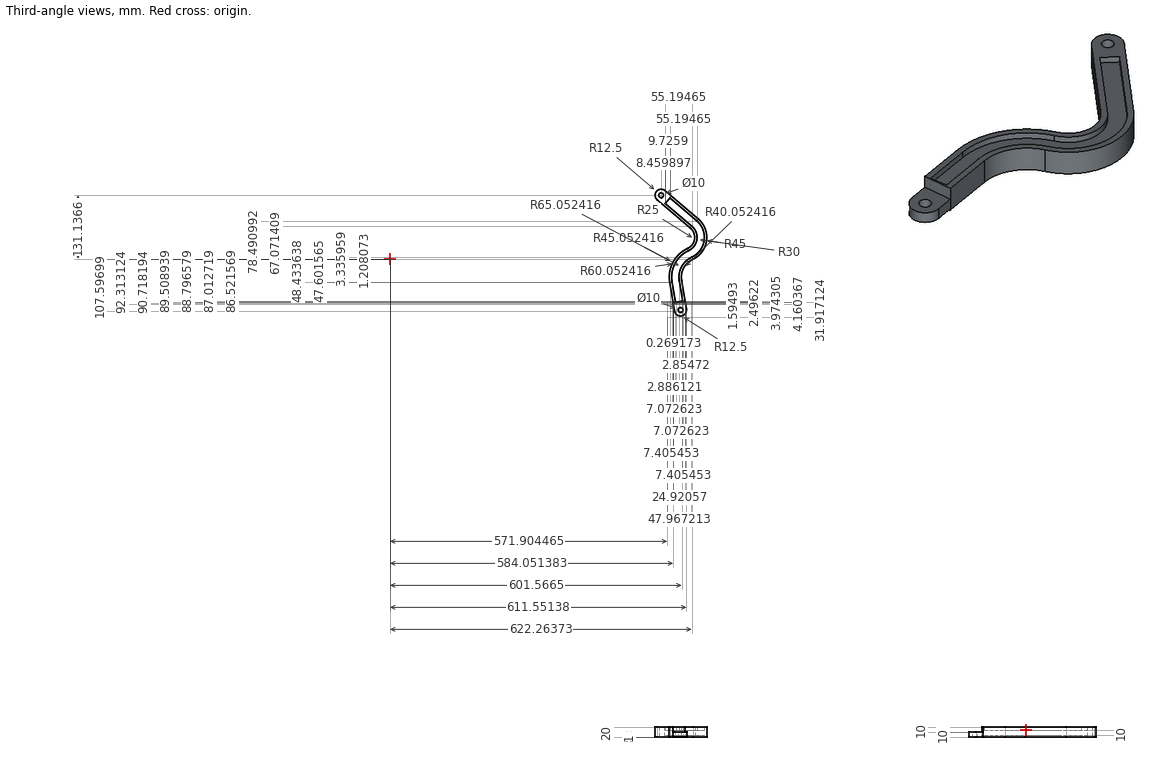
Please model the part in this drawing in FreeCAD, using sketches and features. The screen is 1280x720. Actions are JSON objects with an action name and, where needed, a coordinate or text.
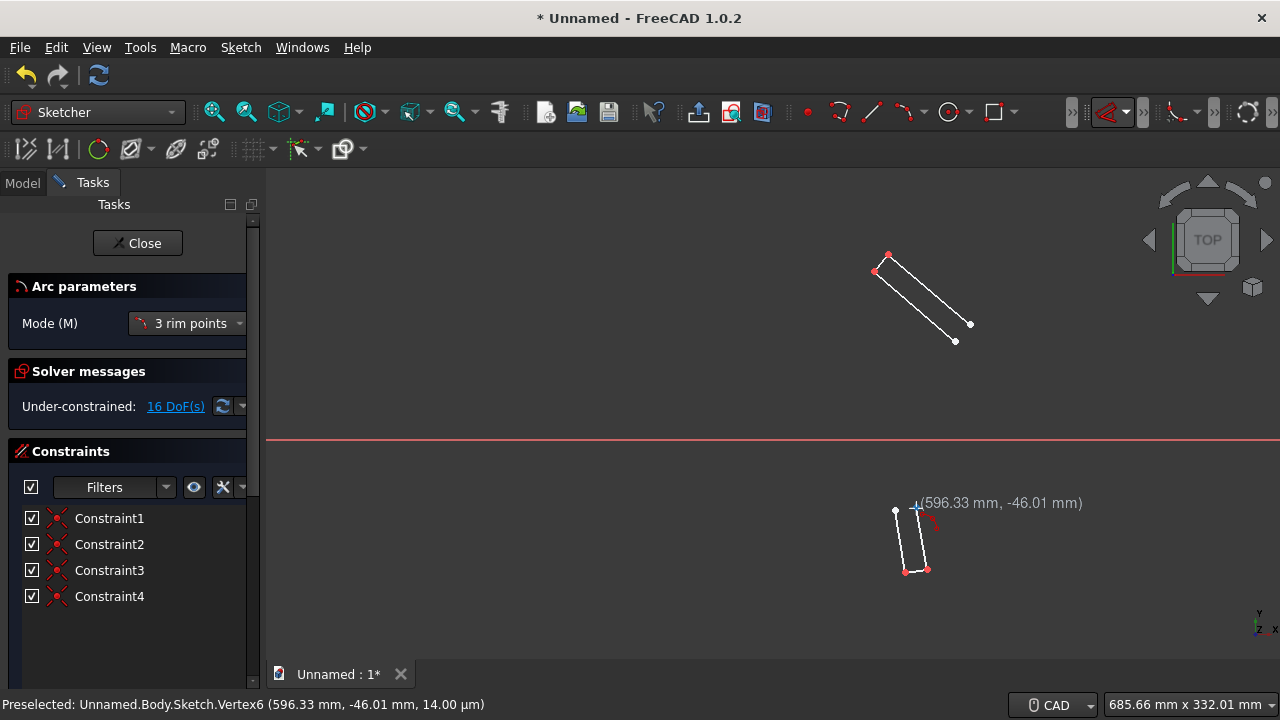
{"action": "scroll", "coordinate": [954, 435], "scroll_direction": "up", "scroll_amount": 6}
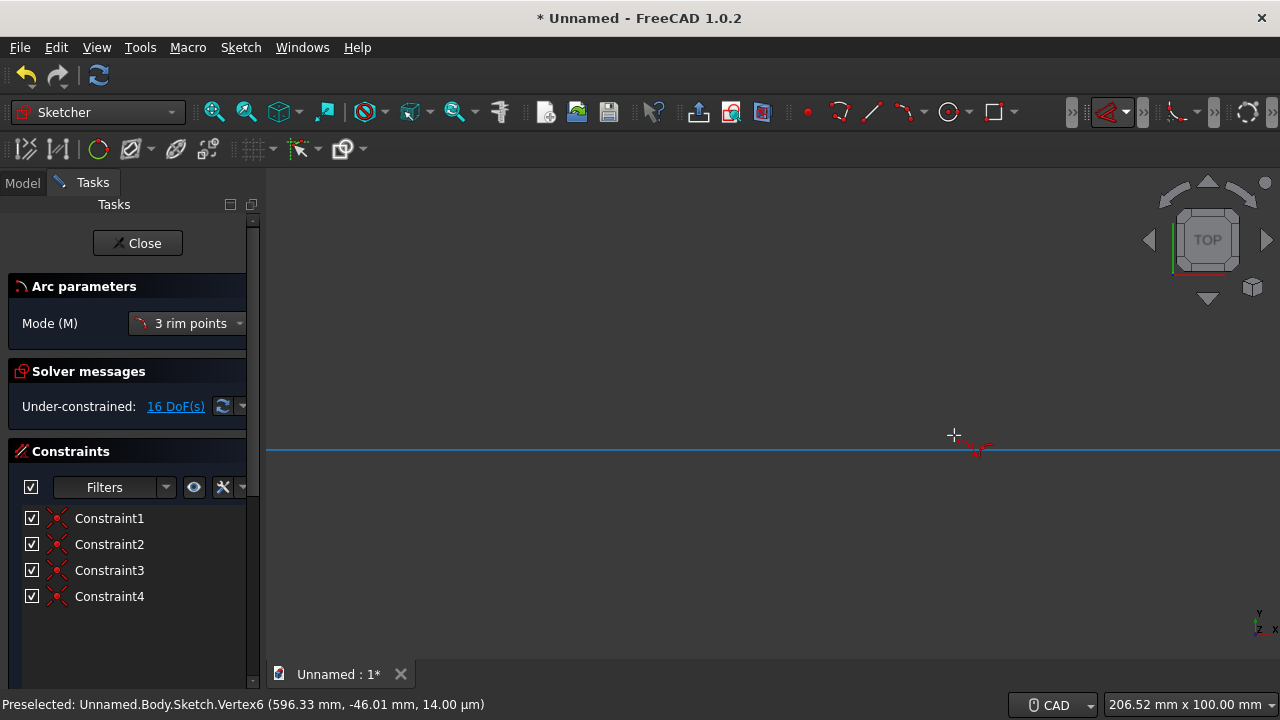
{"action": "left_click", "coordinate": [954, 434]}
{"action": "left_click", "coordinate": [850, 531]}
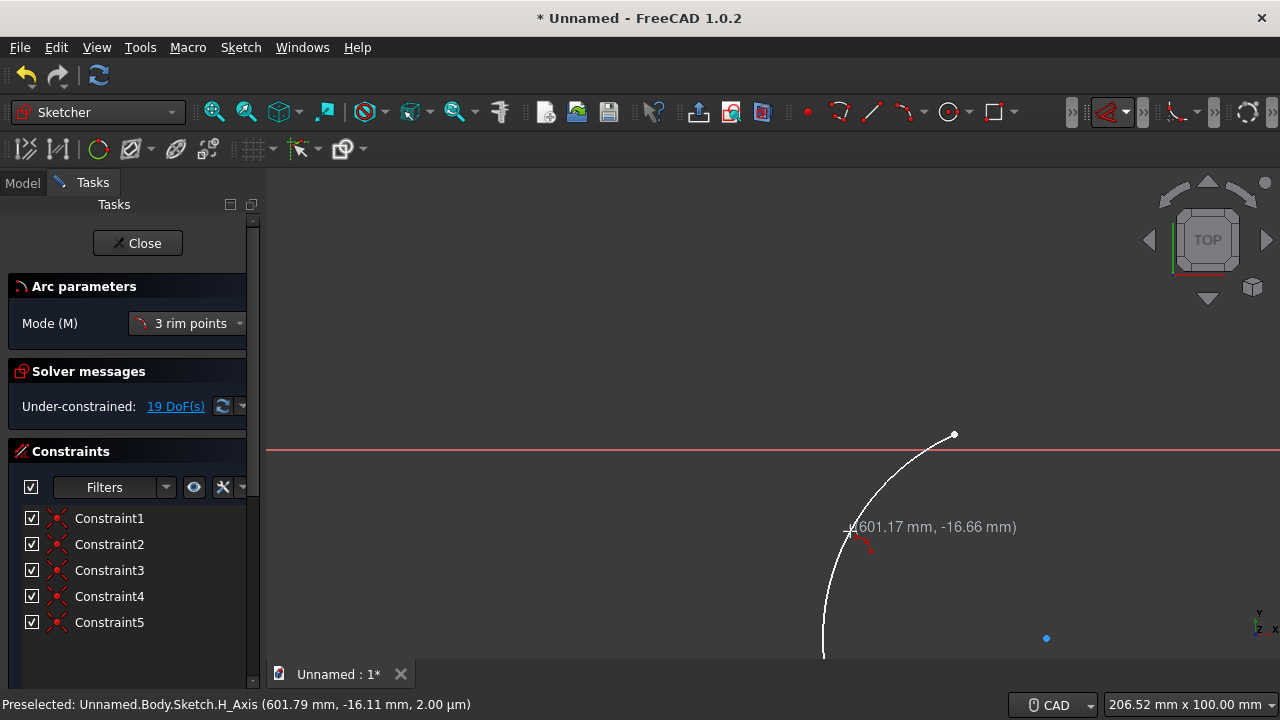
{"action": "left_click", "coordinate": [954, 435]}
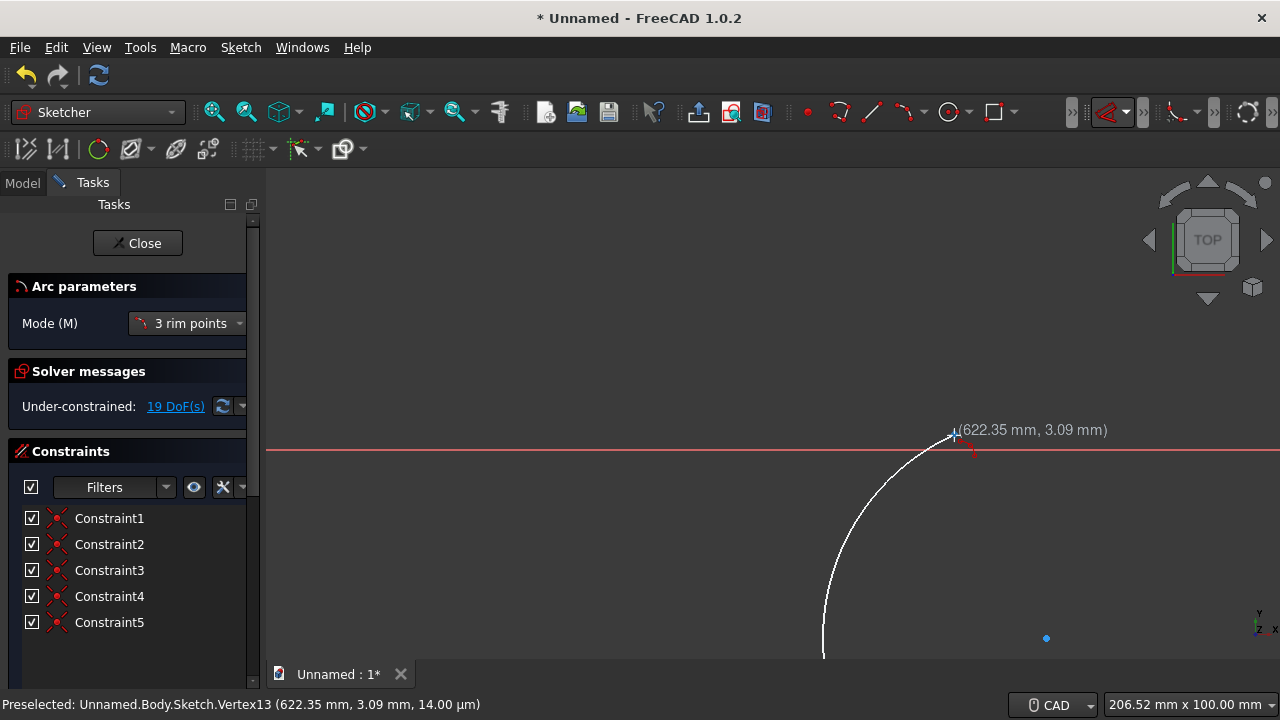
{"action": "scroll", "coordinate": [628, 436], "scroll_direction": "down", "scroll_amount": 6}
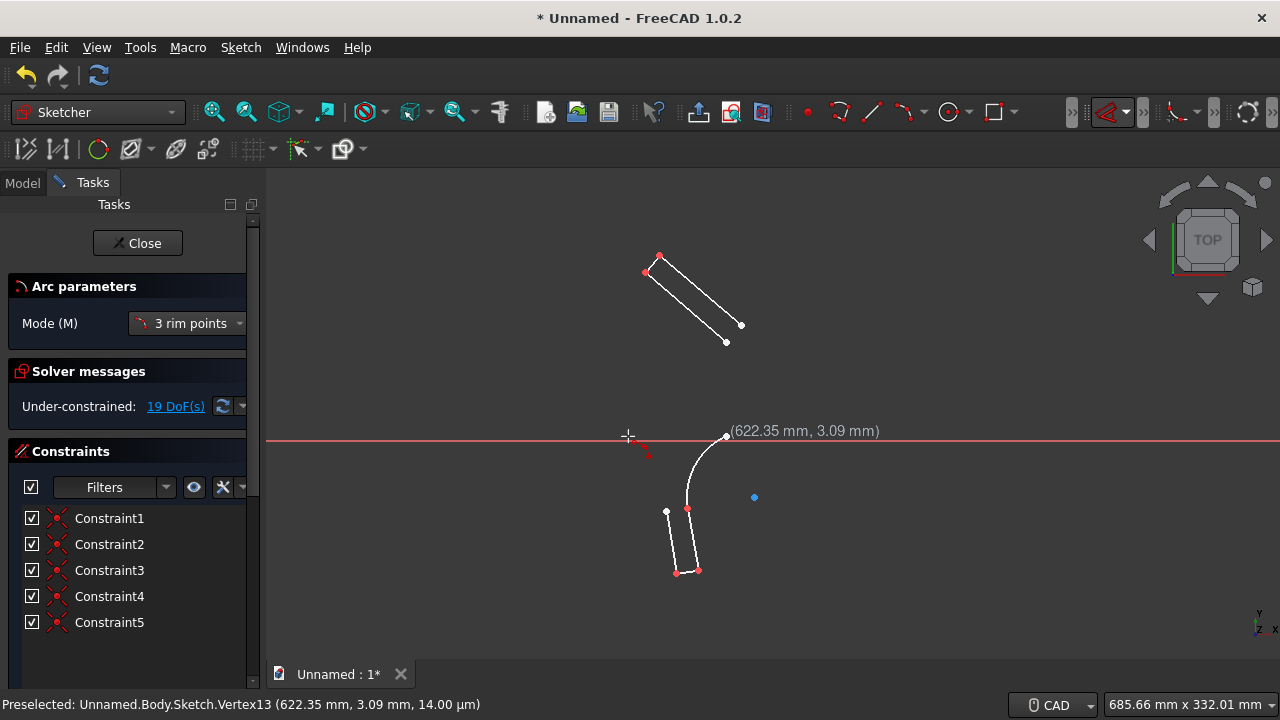
{"action": "left_click", "coordinate": [742, 326]}
{"action": "left_click", "coordinate": [764, 384]}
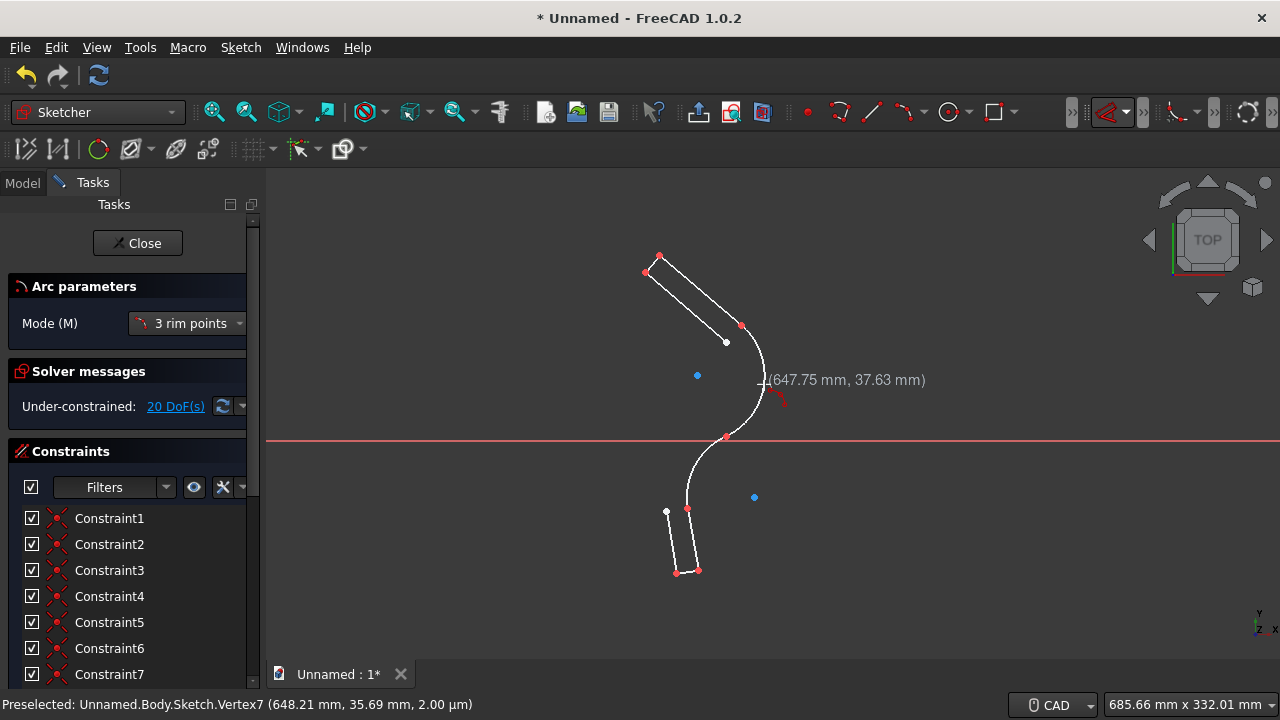
{"action": "left_click", "coordinate": [727, 343]}
{"action": "left_click", "coordinate": [717, 416]}
{"action": "left_click", "coordinate": [742, 381]}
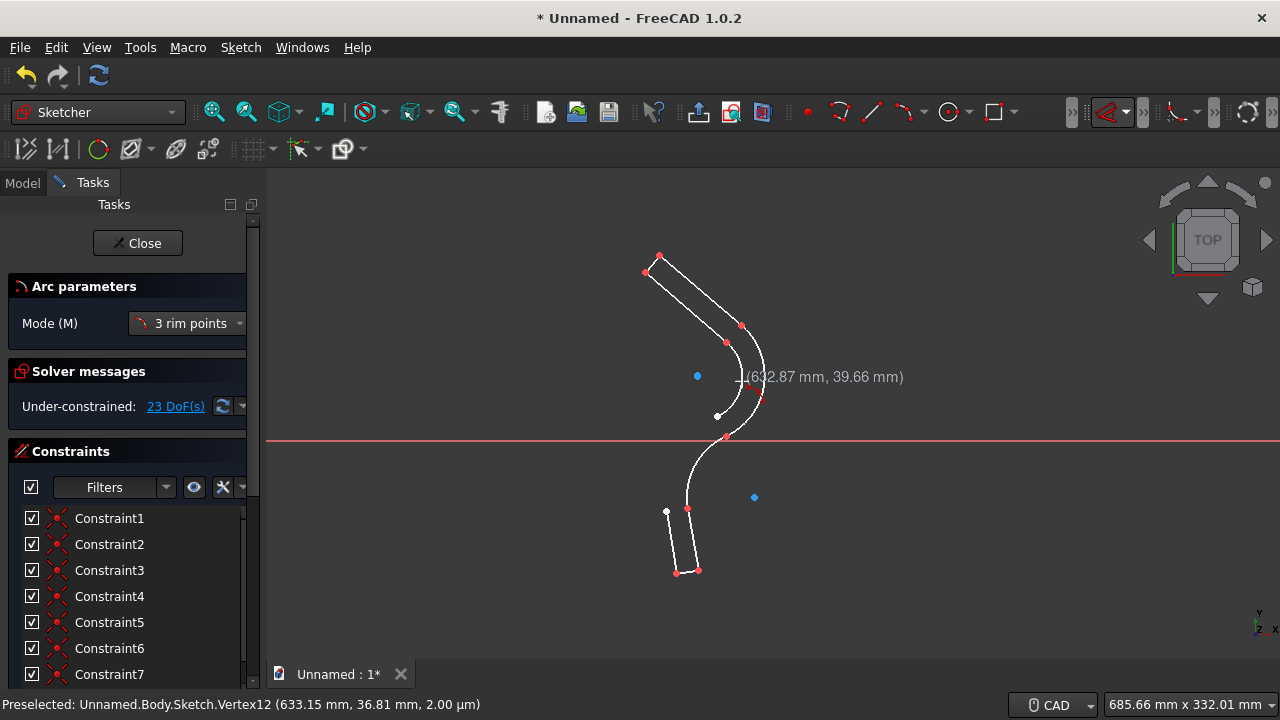
{"action": "left_click", "coordinate": [717, 417]}
{"action": "left_click", "coordinate": [667, 512]}
{"action": "left_click", "coordinate": [676, 455]}
{"action": "key", "text": "Escape"}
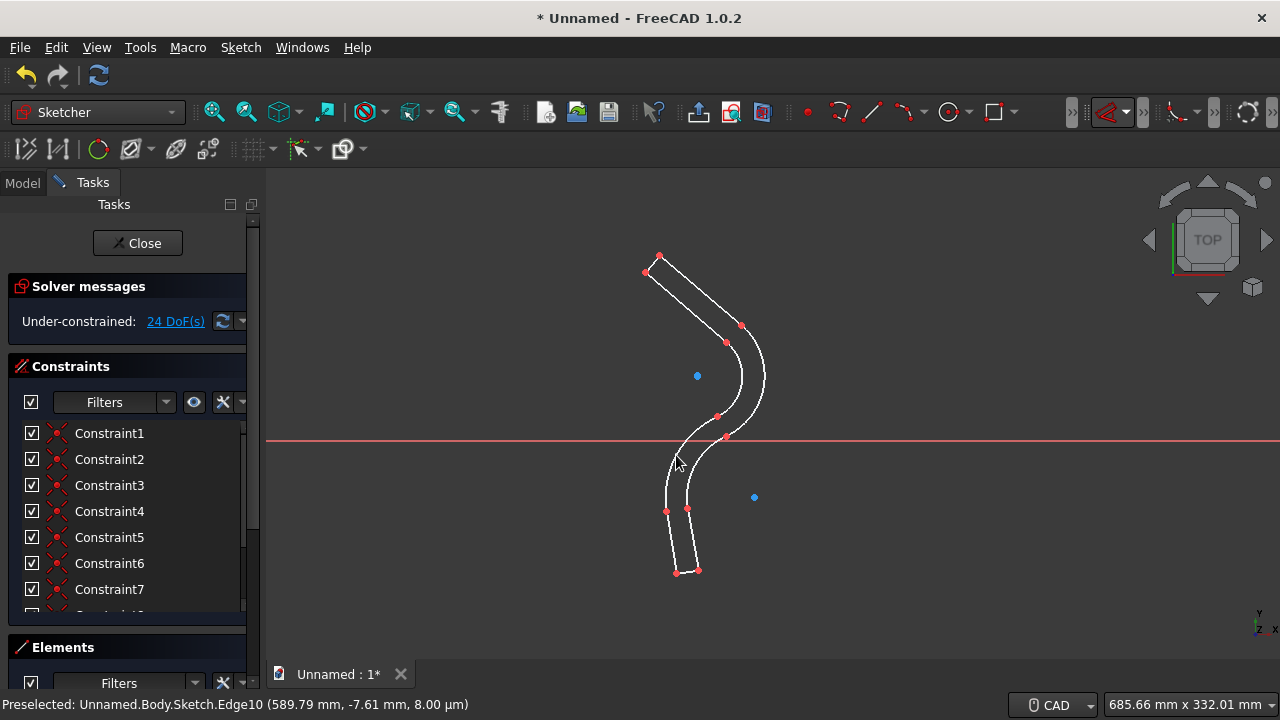
{"action": "left_click", "coordinate": [670, 530]}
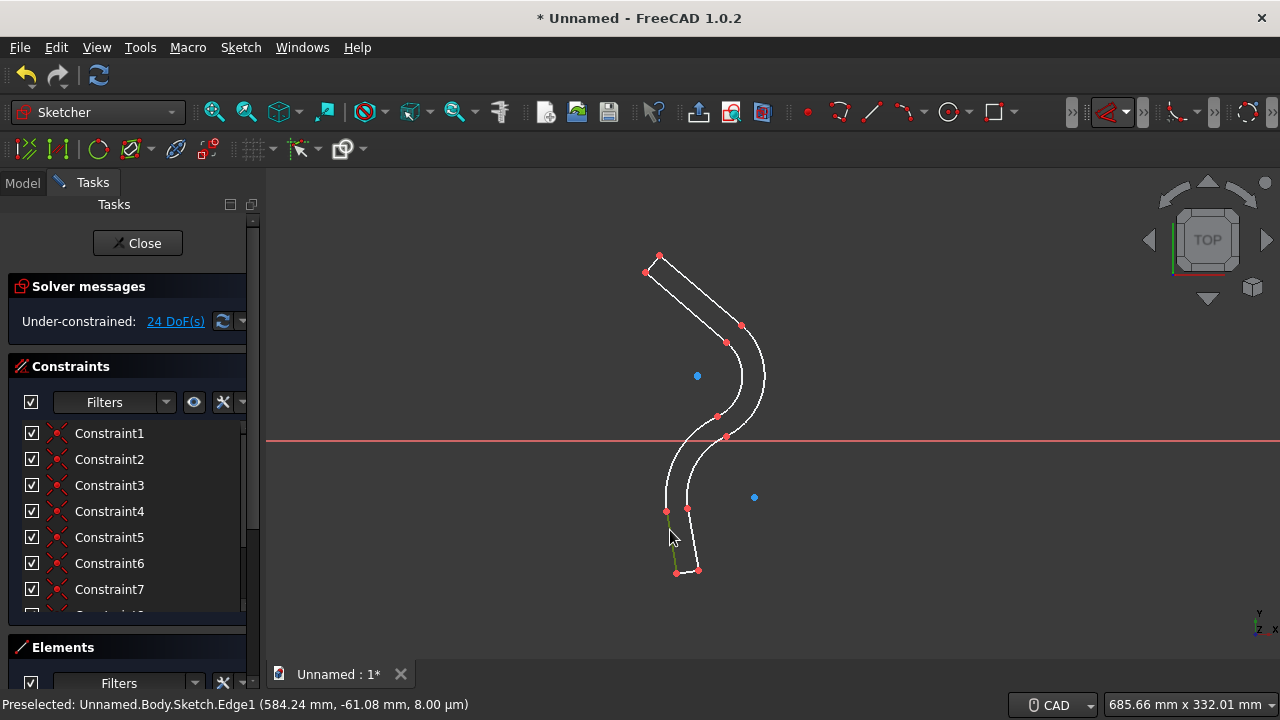
{"action": "left_click", "coordinate": [689, 437]}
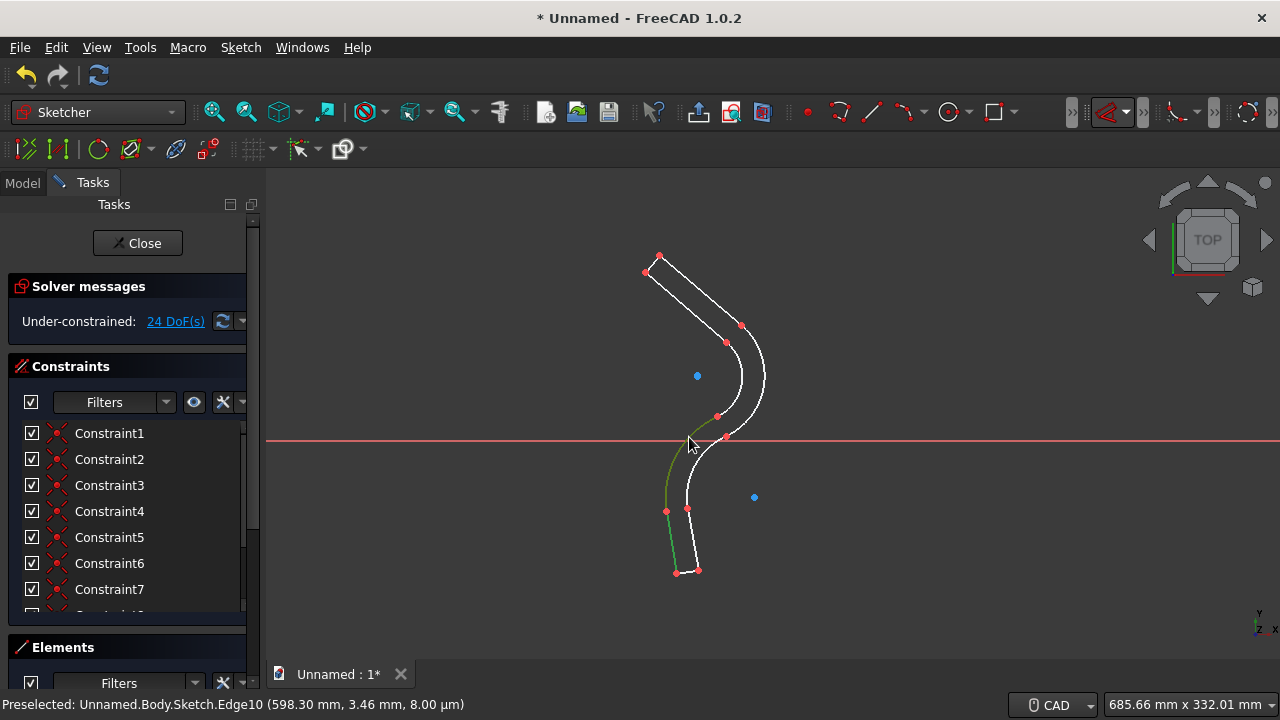
{"action": "key", "text": "t"}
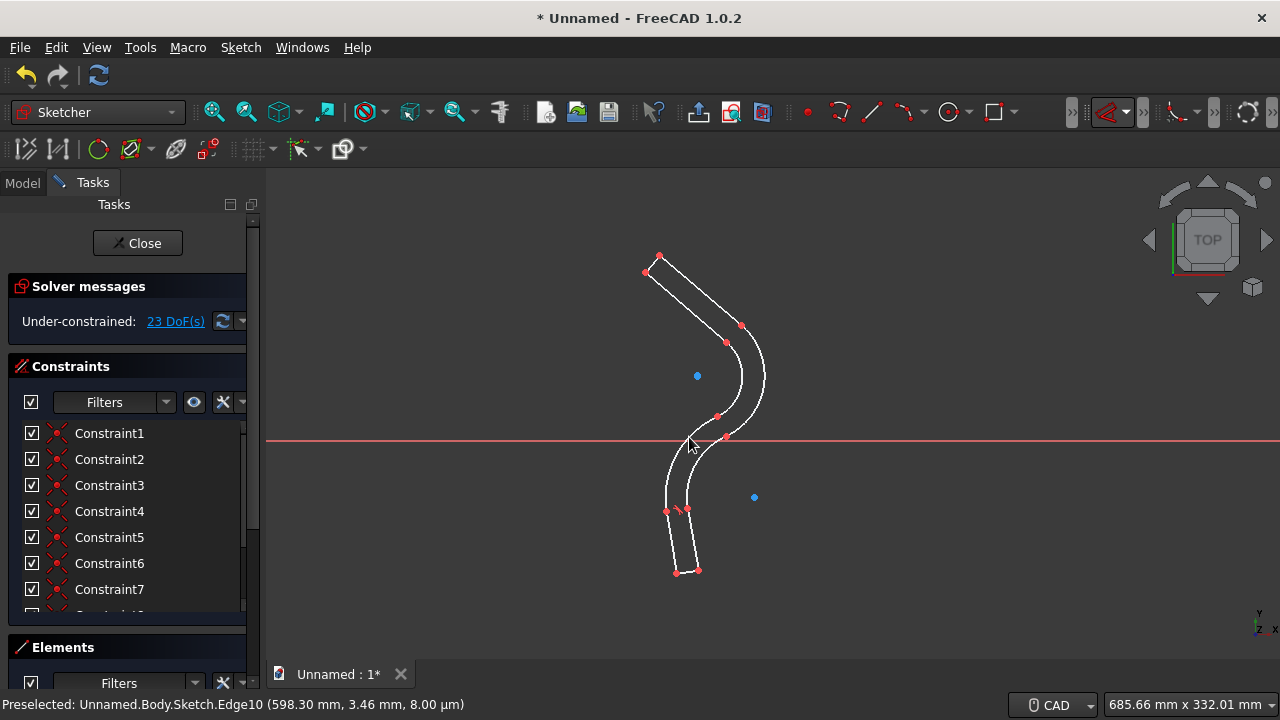
{"action": "left_click", "coordinate": [696, 552]}